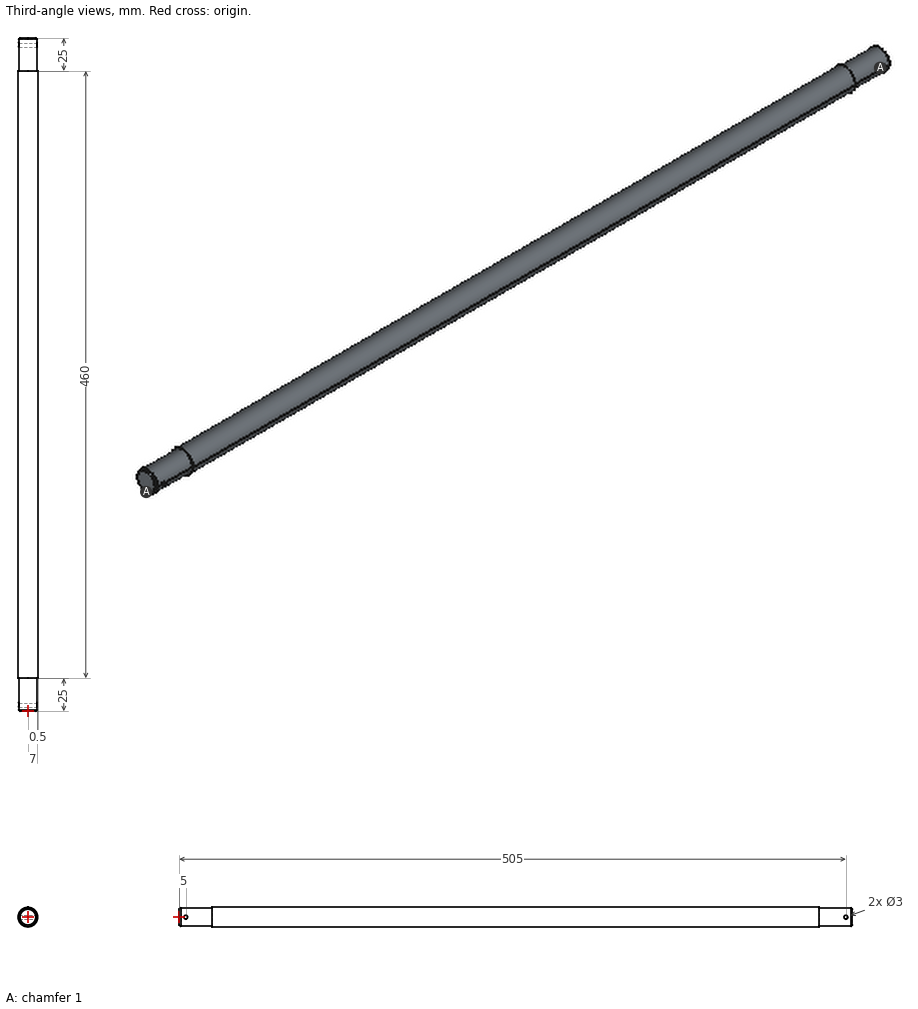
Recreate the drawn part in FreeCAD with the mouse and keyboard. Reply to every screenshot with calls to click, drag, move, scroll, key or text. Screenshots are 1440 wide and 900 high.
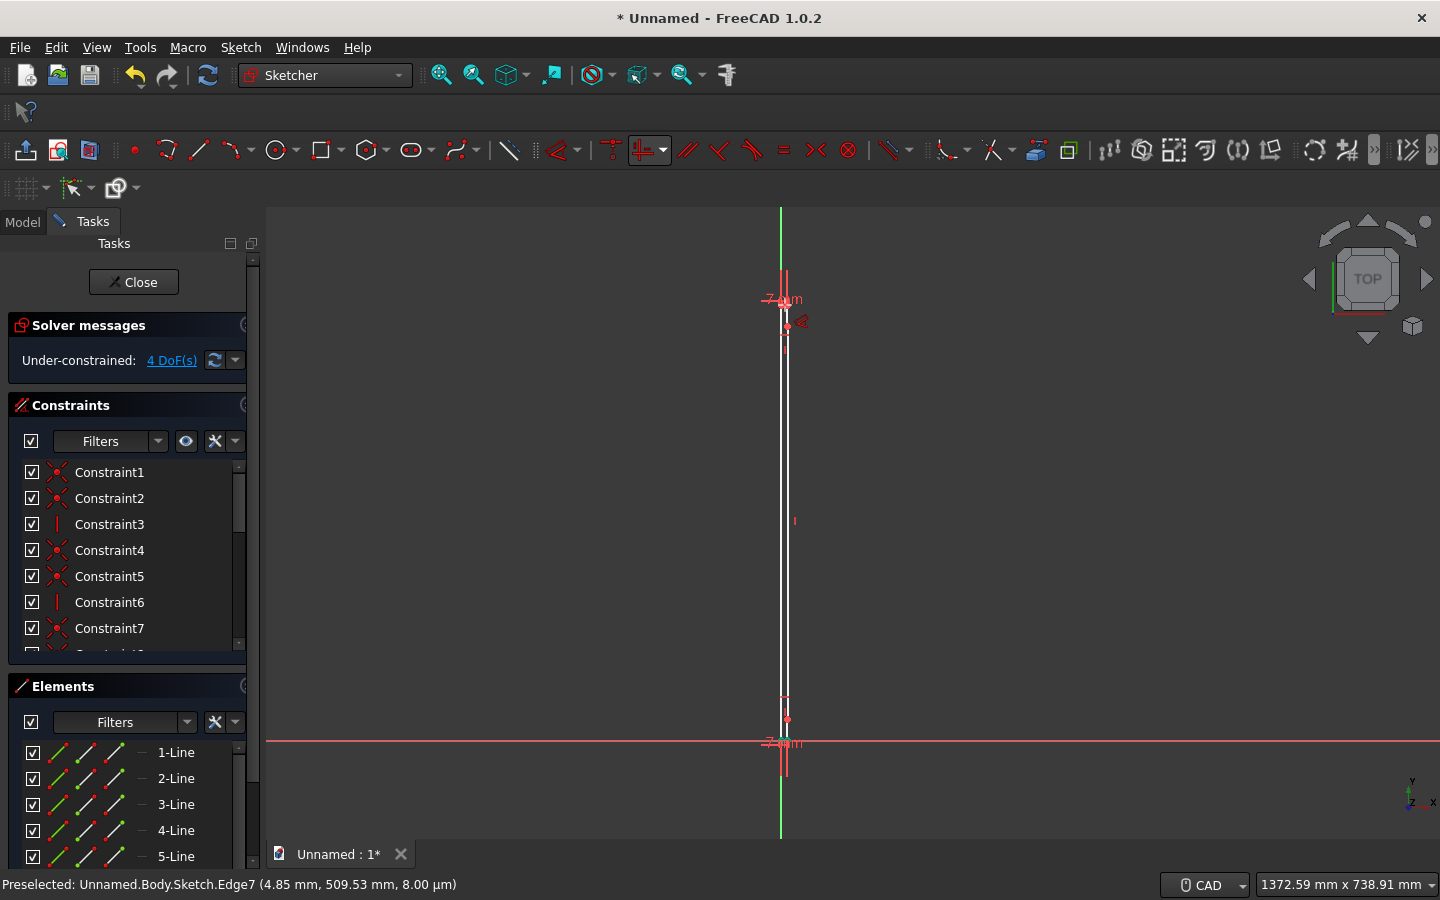
scroll(787, 735, up, 5)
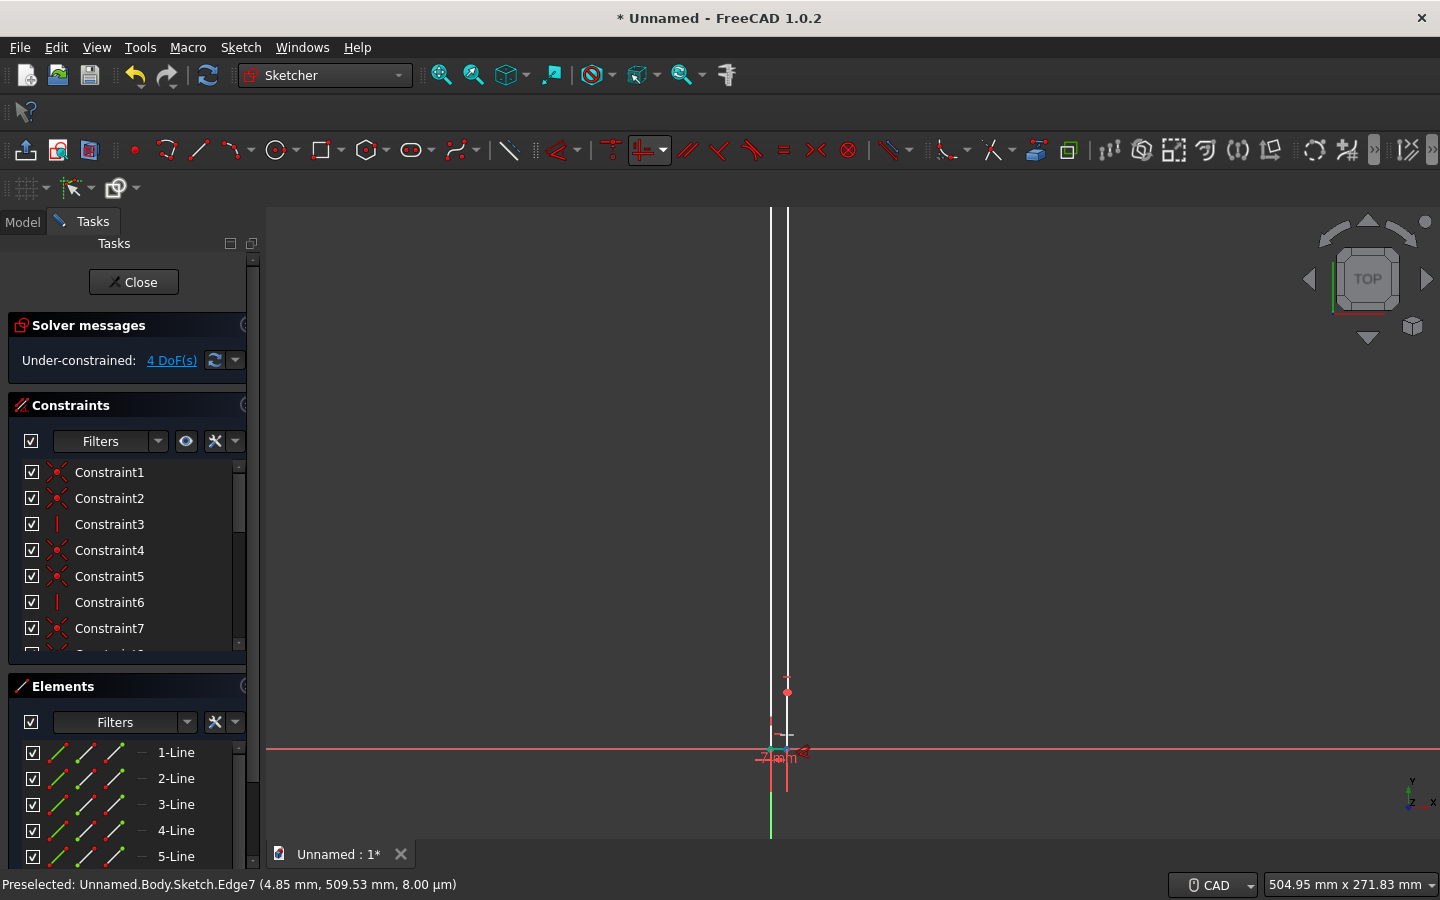
click(787, 732)
click(821, 721)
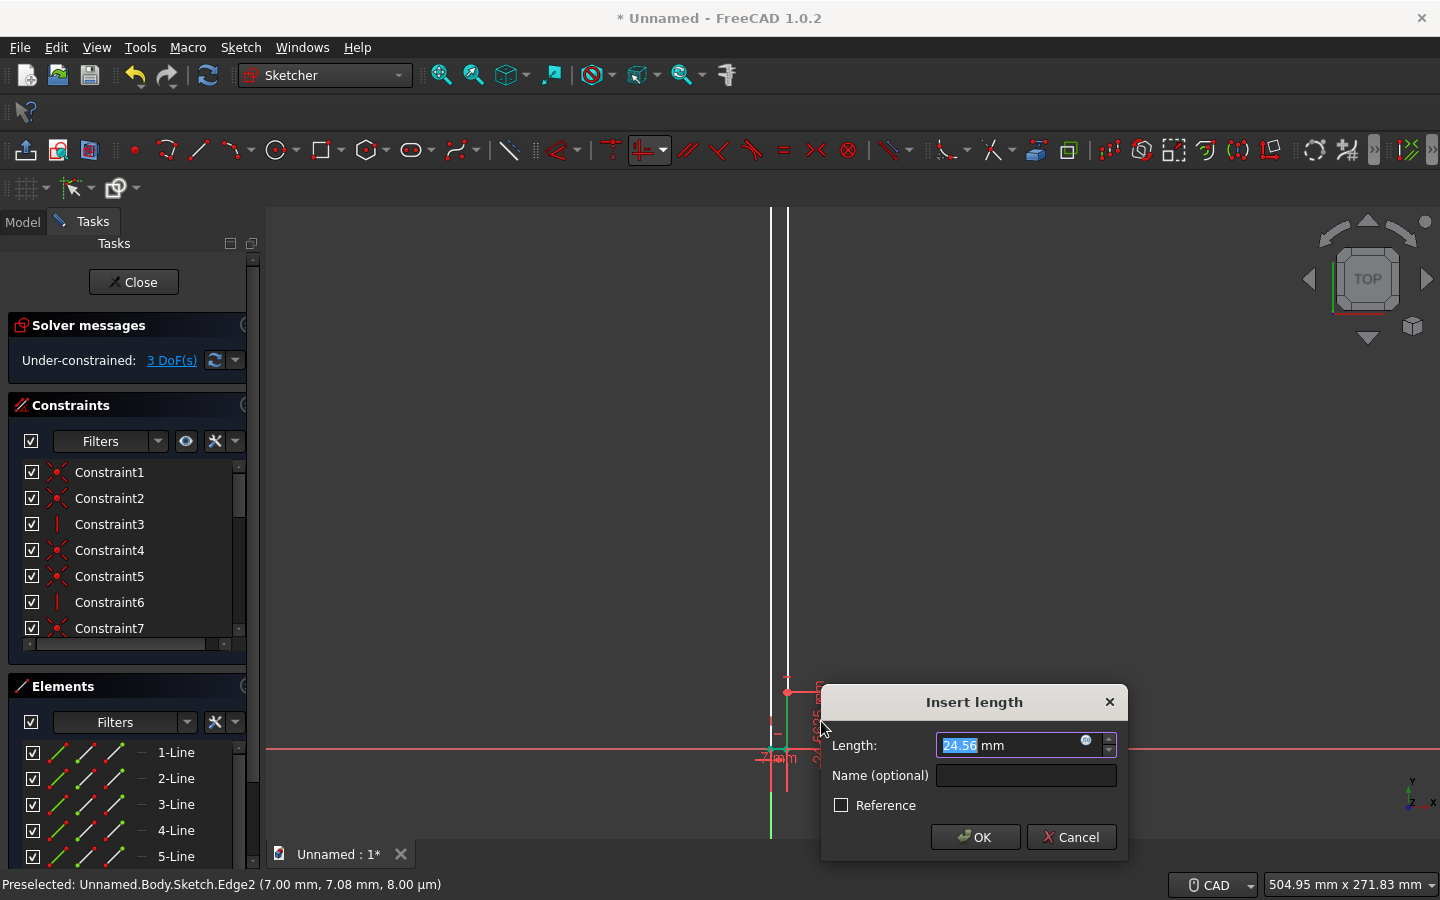
text(25)
key(Return)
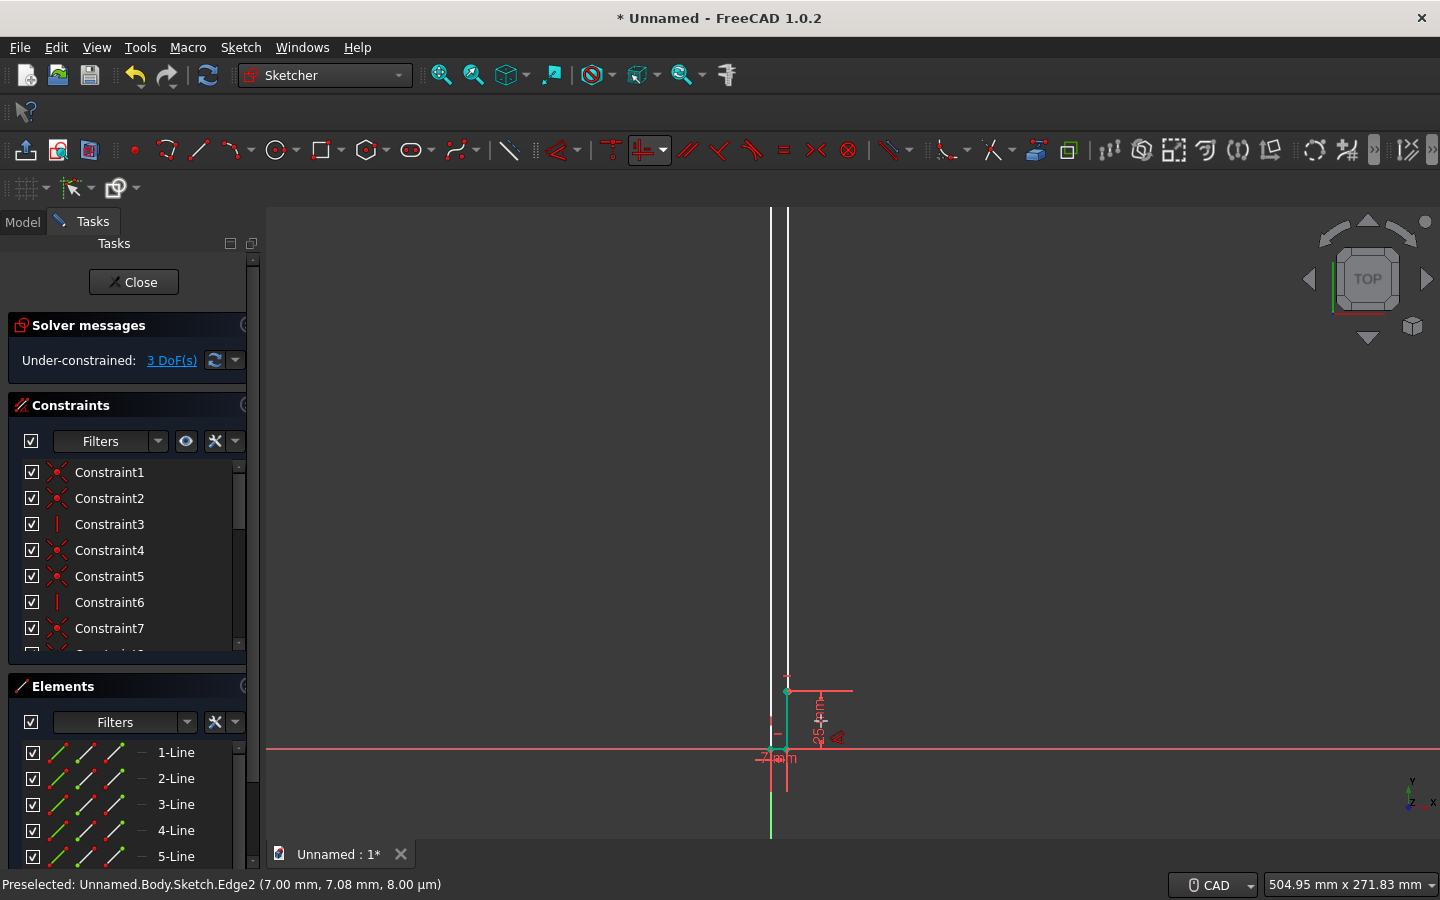
scroll(788, 736, down, 5)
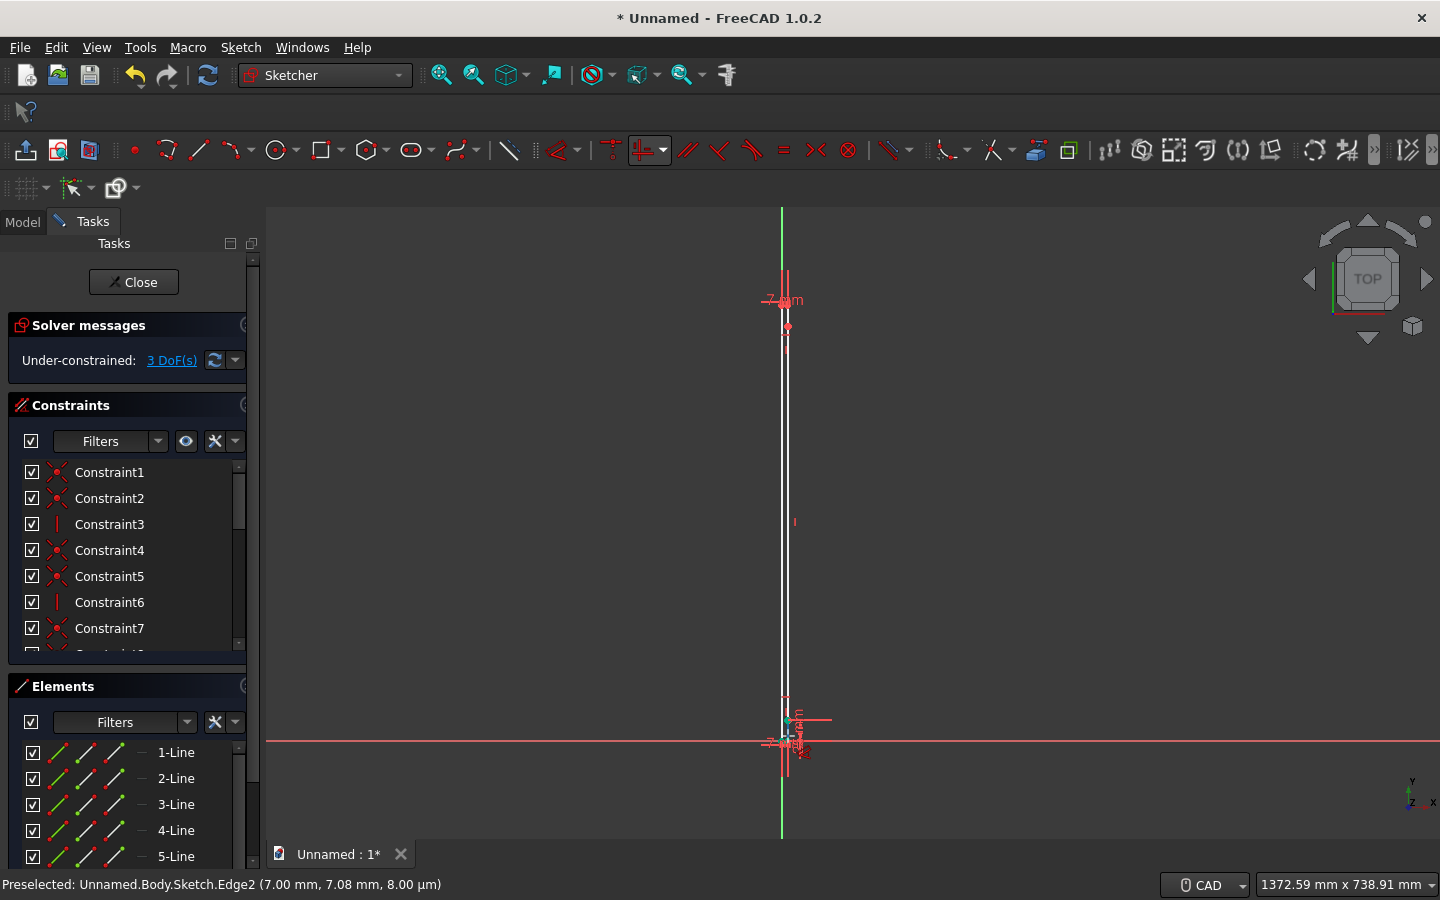
scroll(788, 321, up, 5)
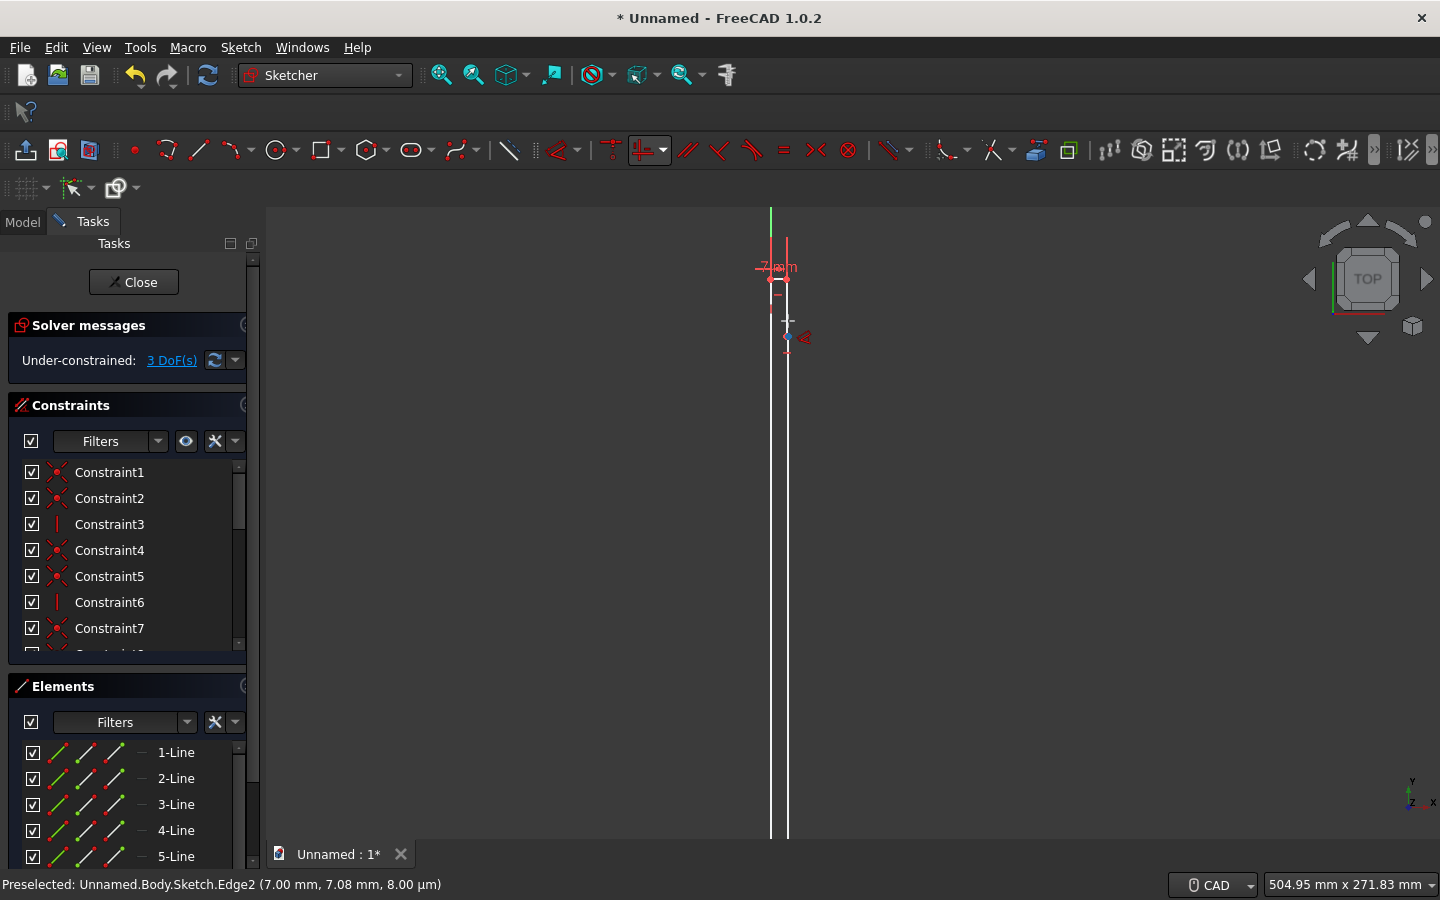
click(787, 320)
click(821, 308)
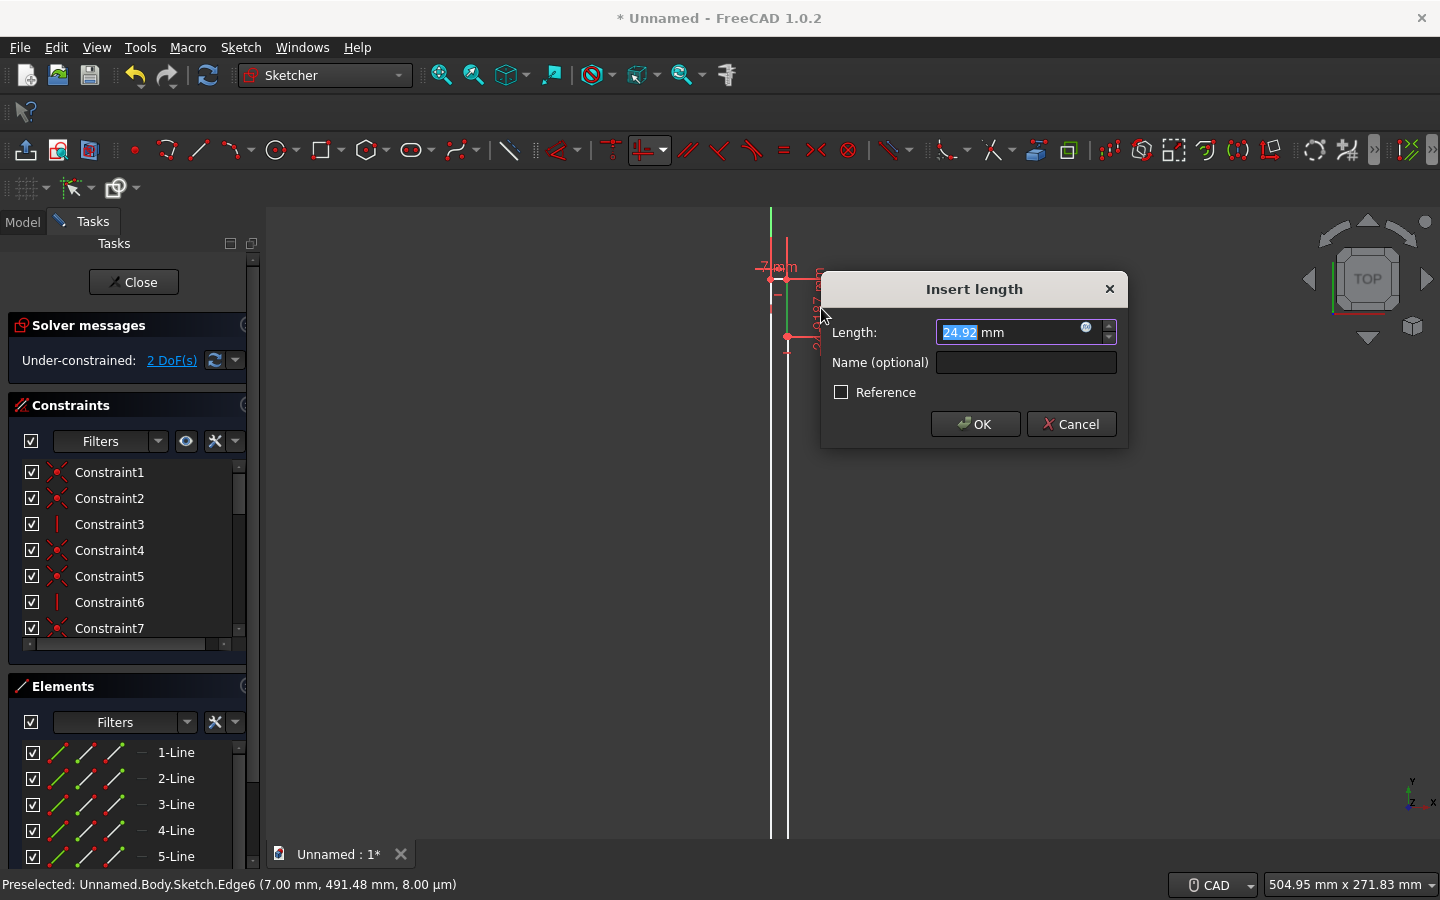
text(25)
key(Return)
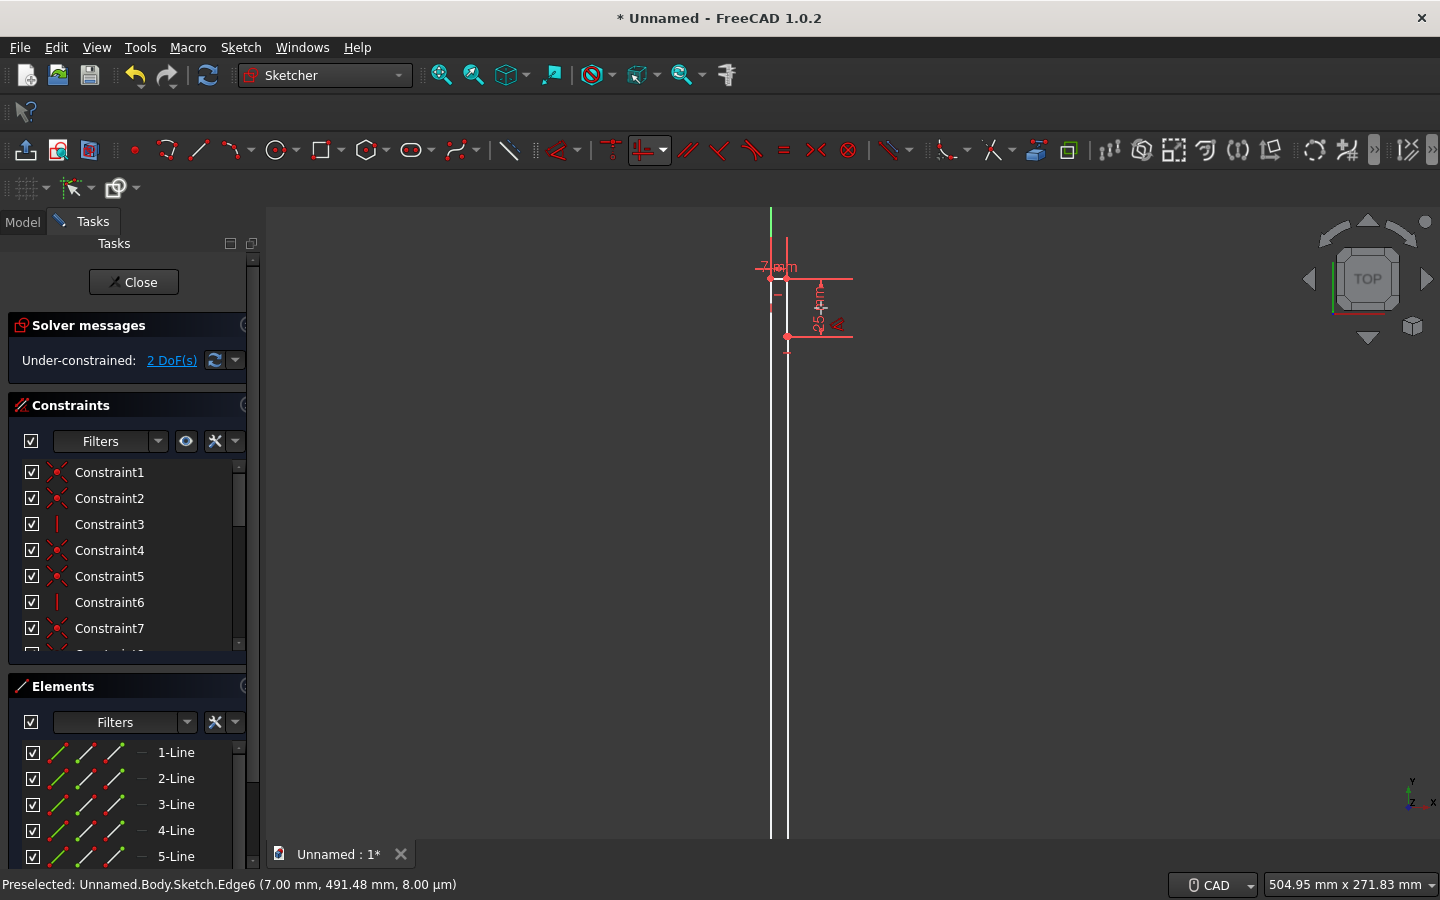
scroll(788, 321, down, 5)